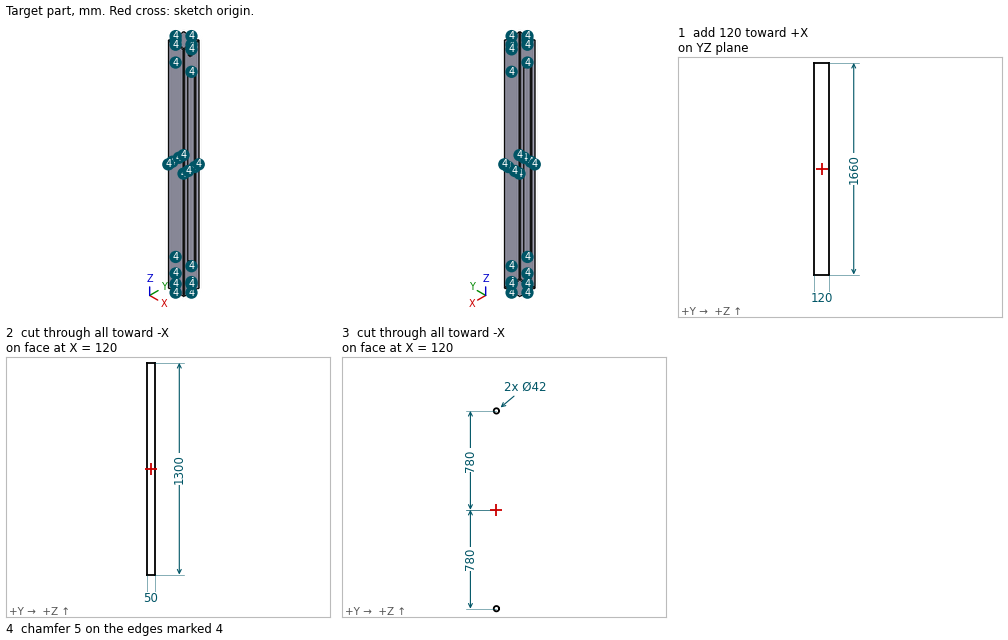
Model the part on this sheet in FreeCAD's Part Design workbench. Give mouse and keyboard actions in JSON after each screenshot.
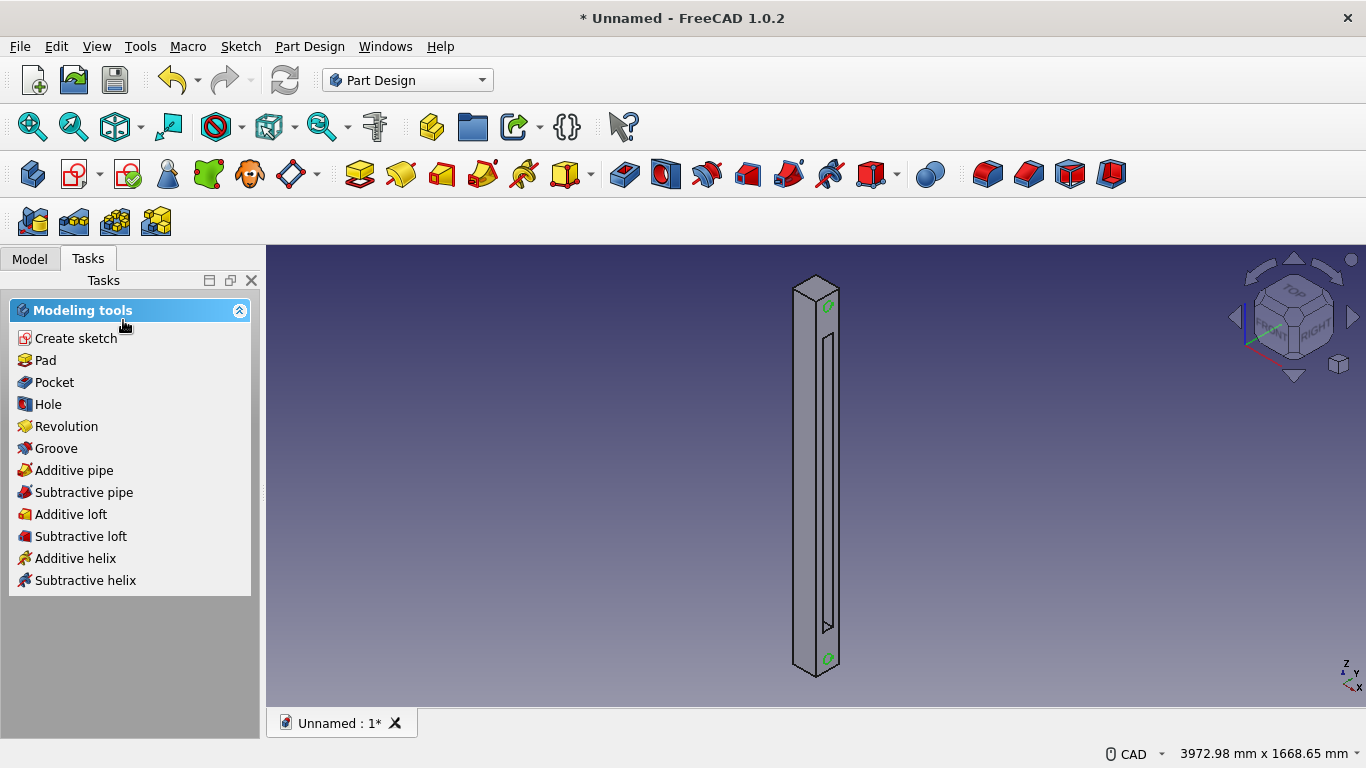
{"action": "left_click", "coordinate": [625, 174]}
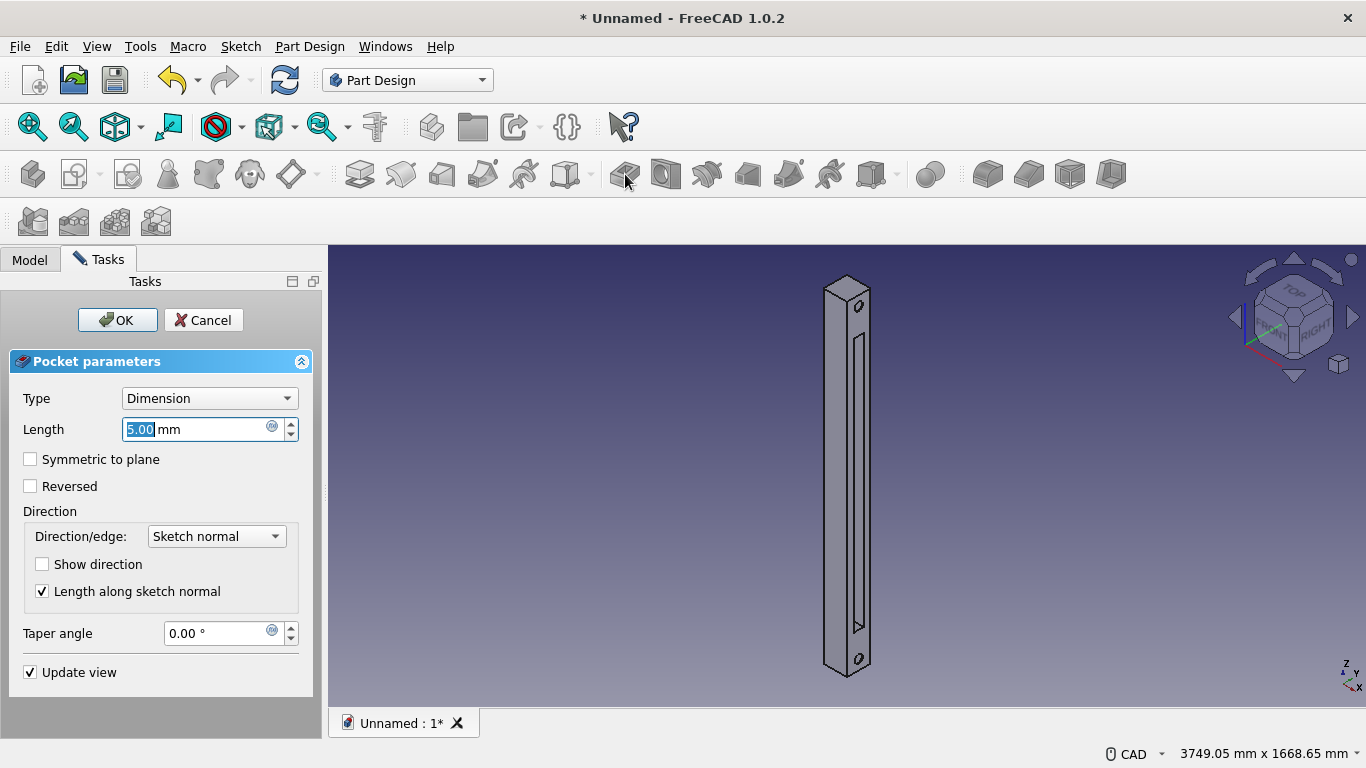
{"action": "left_click", "coordinate": [210, 398]}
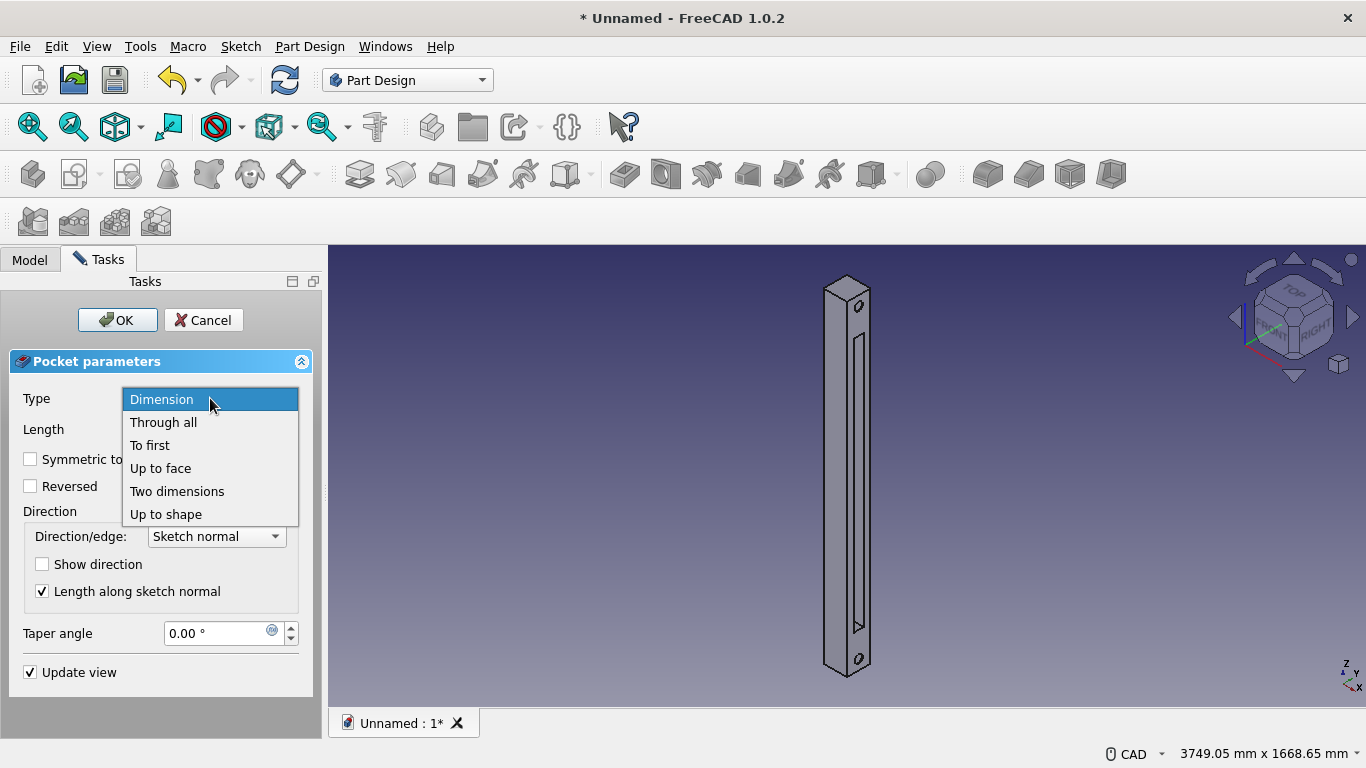
{"action": "left_click", "coordinate": [208, 422]}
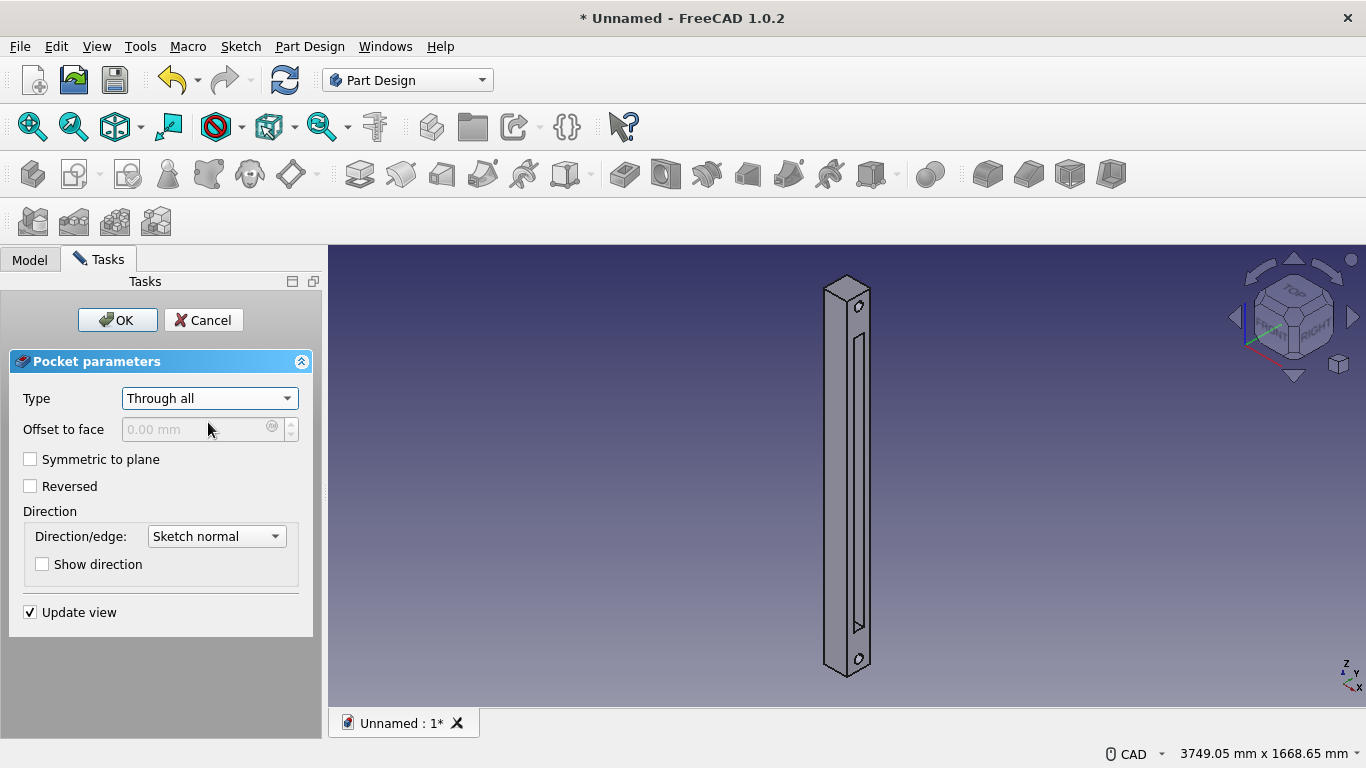
{"action": "left_click", "coordinate": [118, 320]}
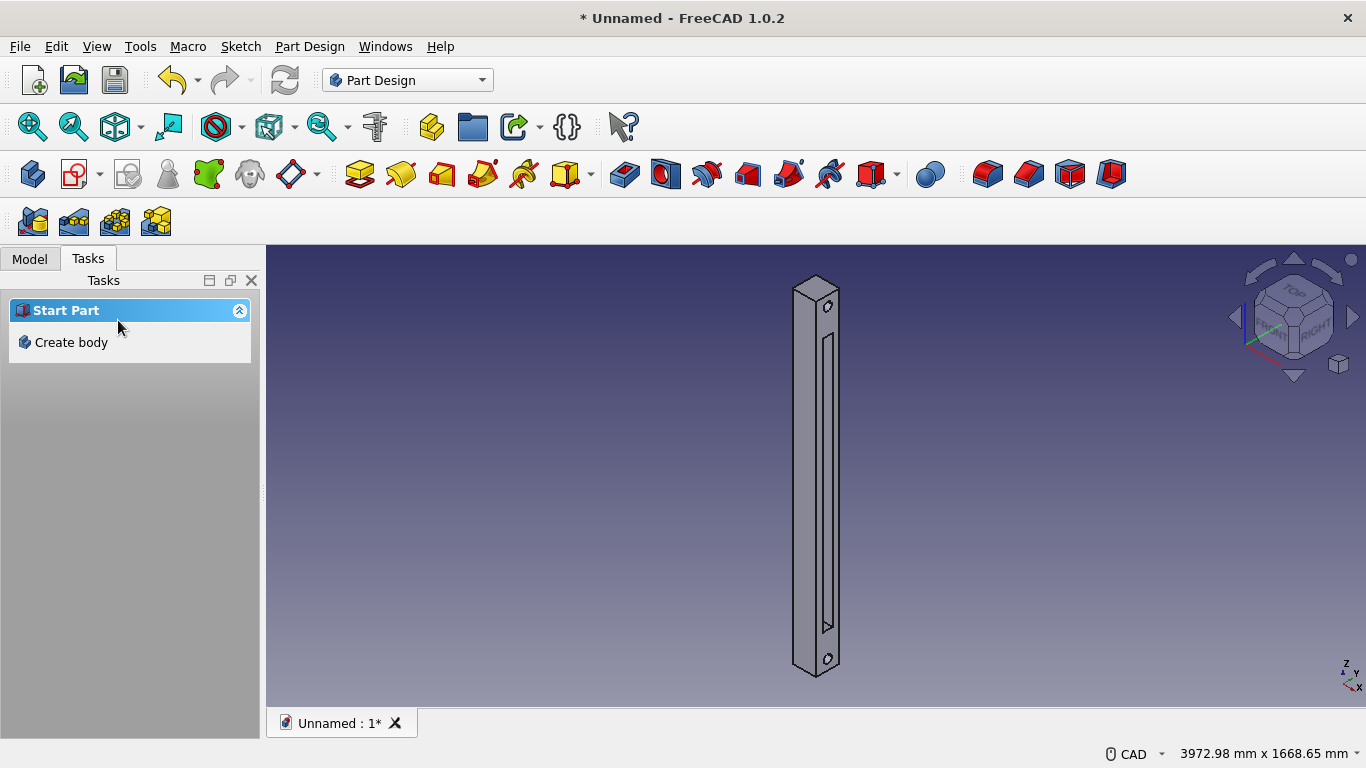
{"action": "left_click", "coordinate": [804, 643]}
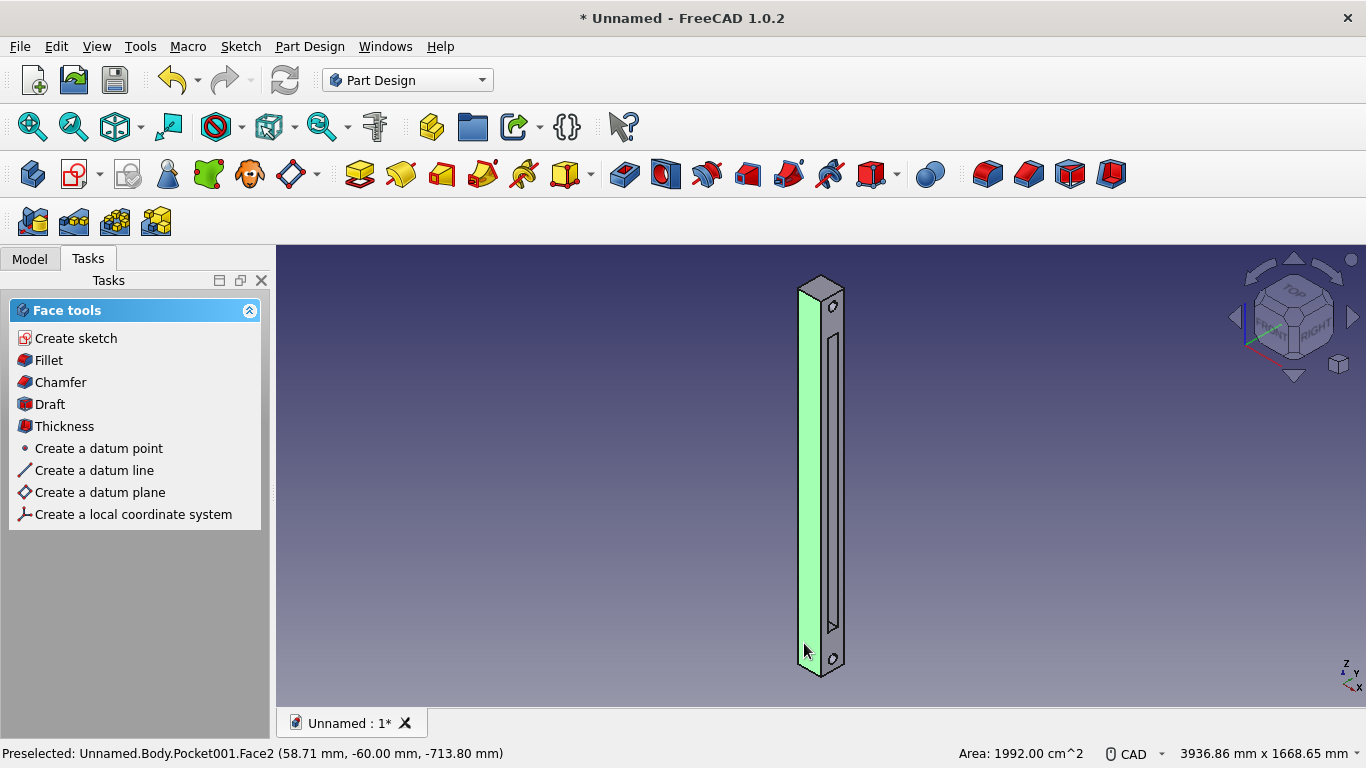
{"action": "left_click", "coordinate": [833, 321], "text": "ctrl"}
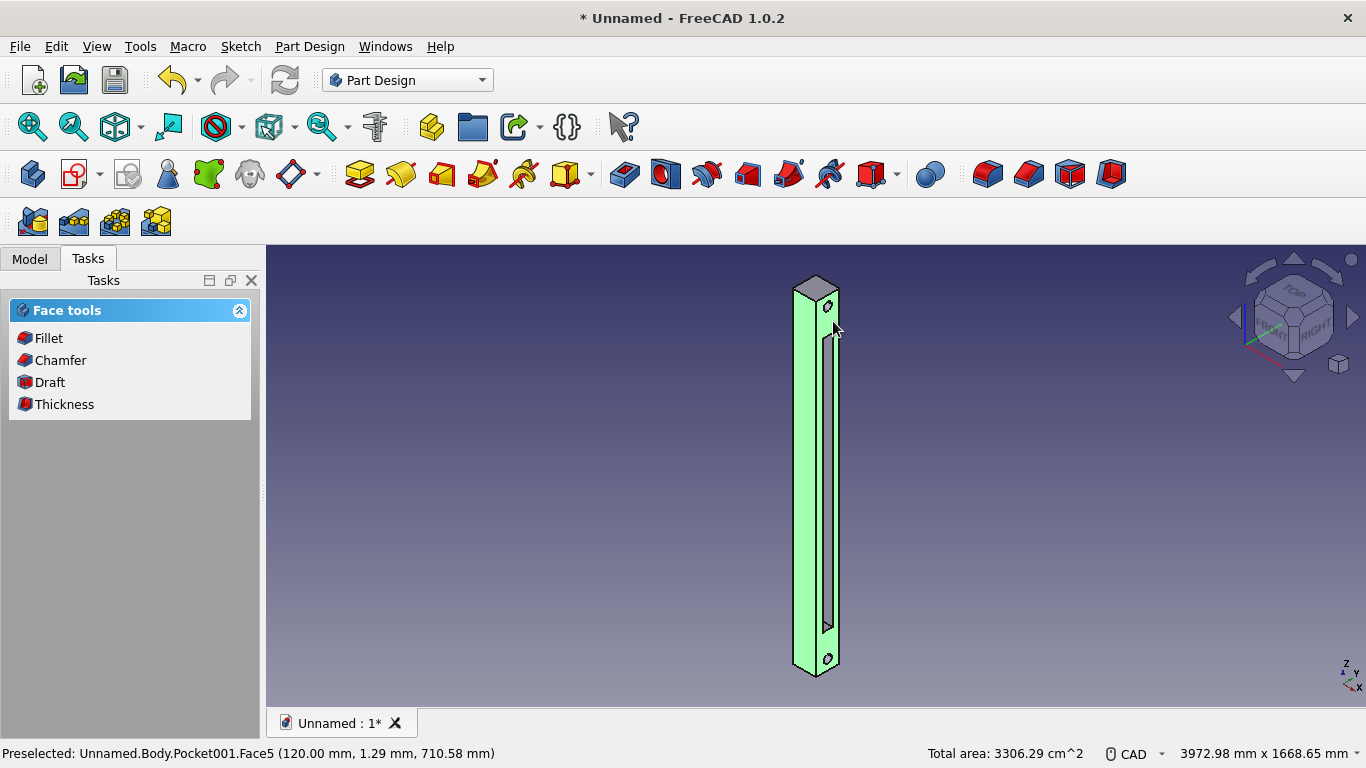
{"action": "key", "text": "2"}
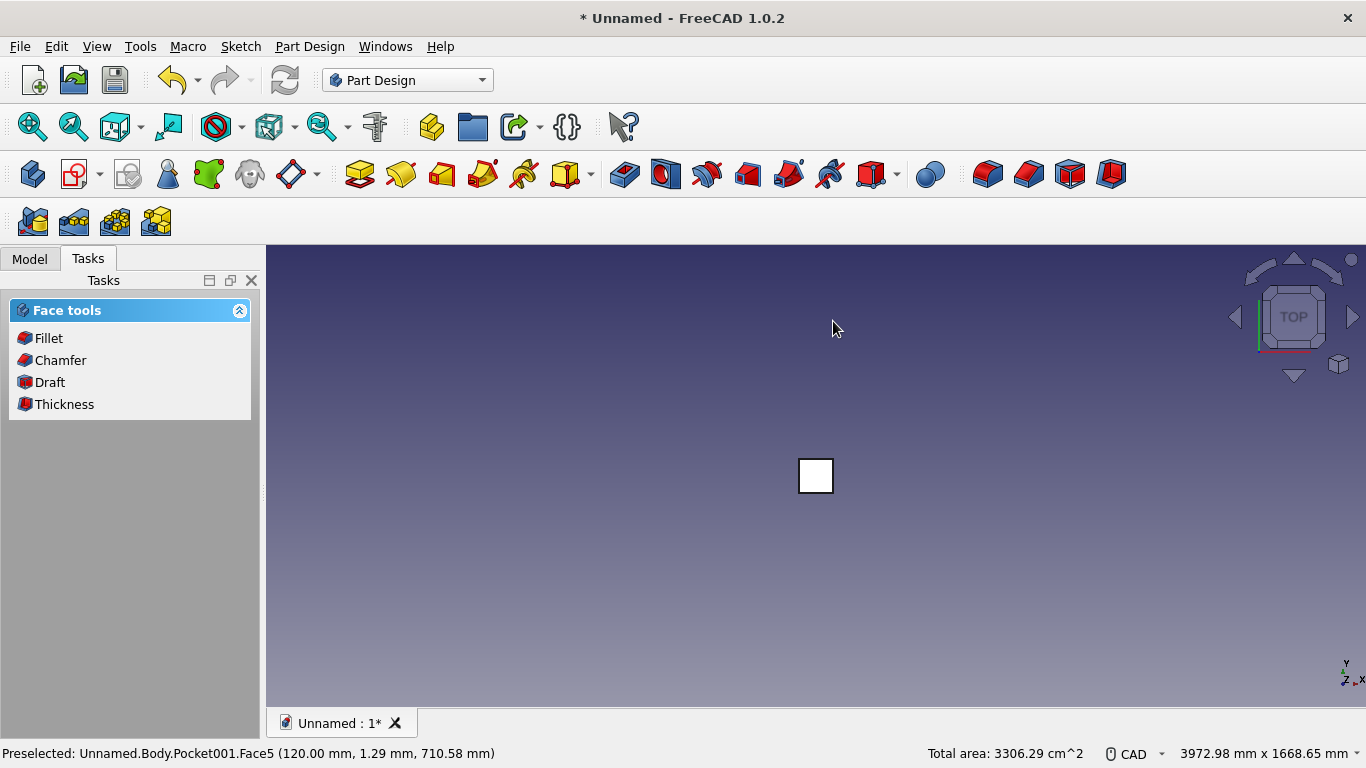
{"action": "key", "text": "v f"}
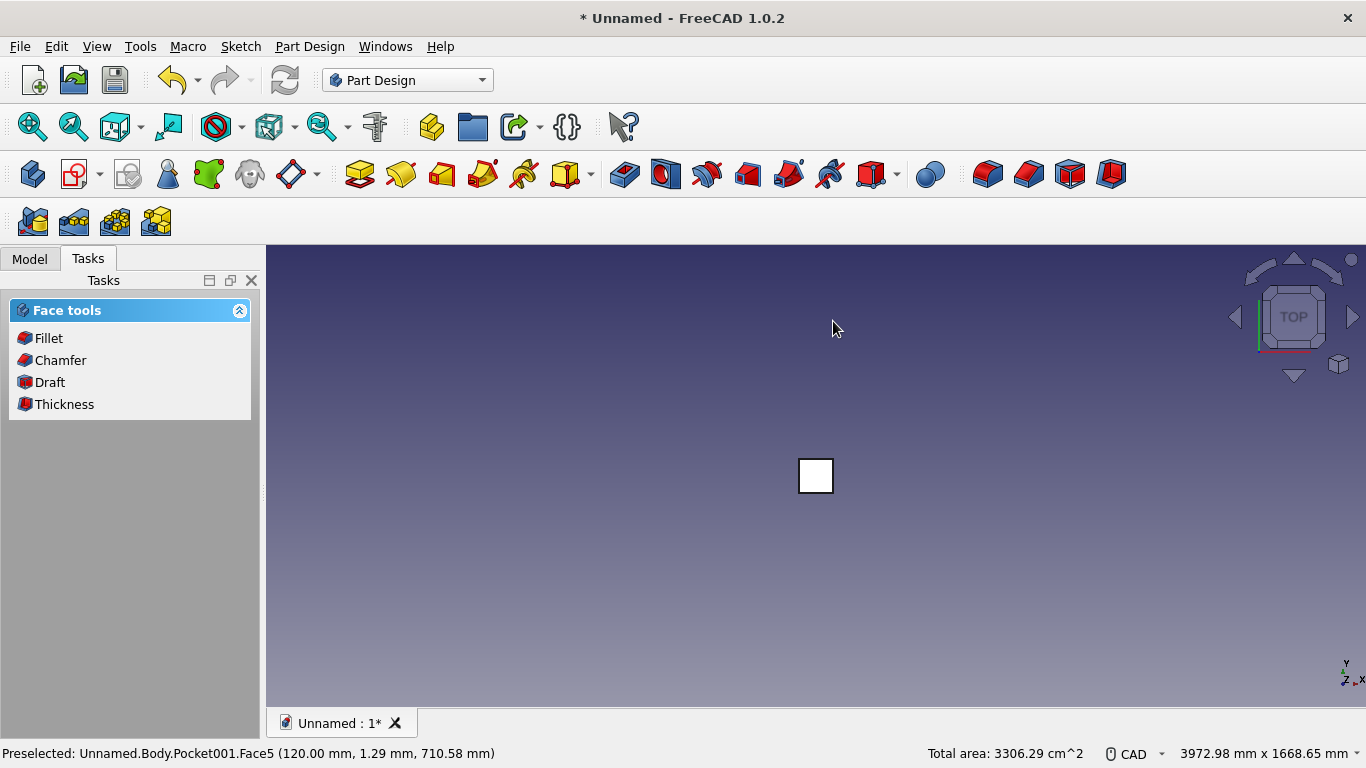
{"action": "key", "text": "0"}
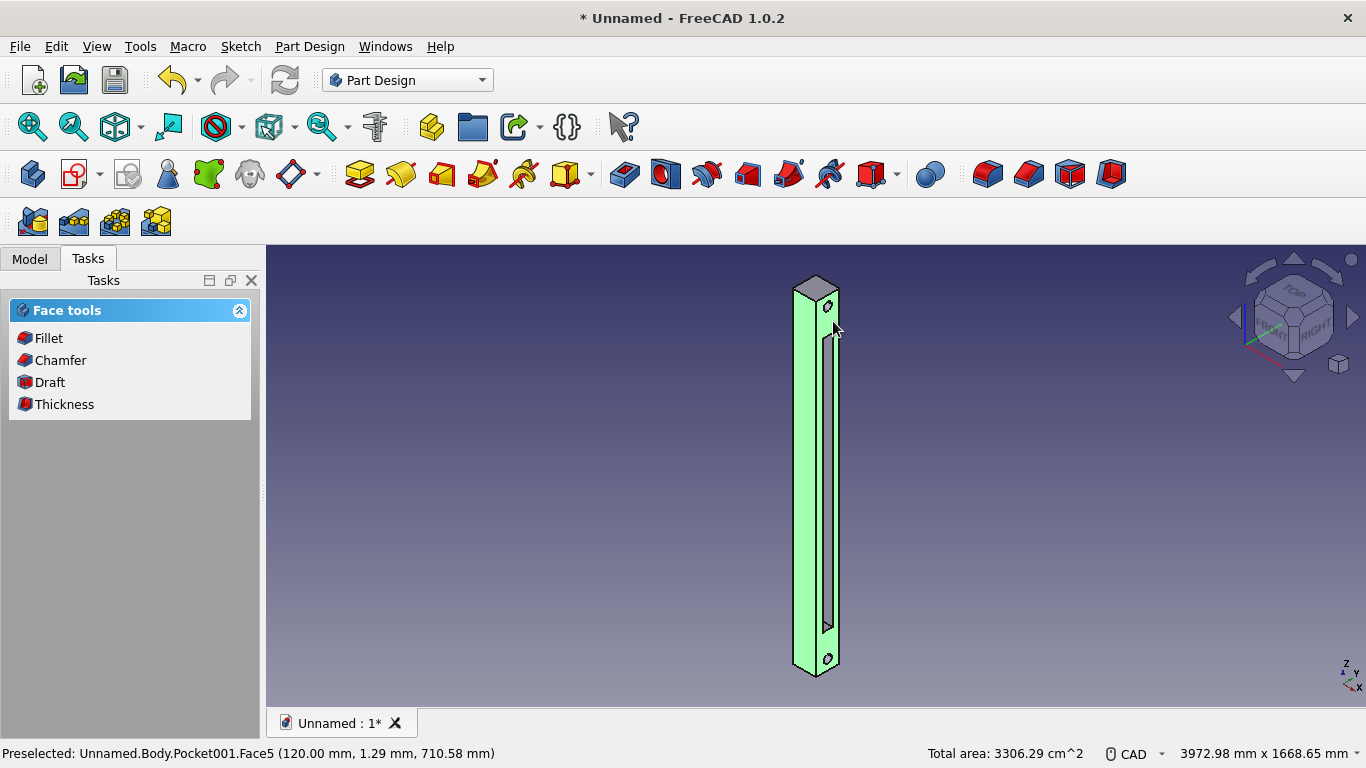
{"action": "key", "text": "1"}